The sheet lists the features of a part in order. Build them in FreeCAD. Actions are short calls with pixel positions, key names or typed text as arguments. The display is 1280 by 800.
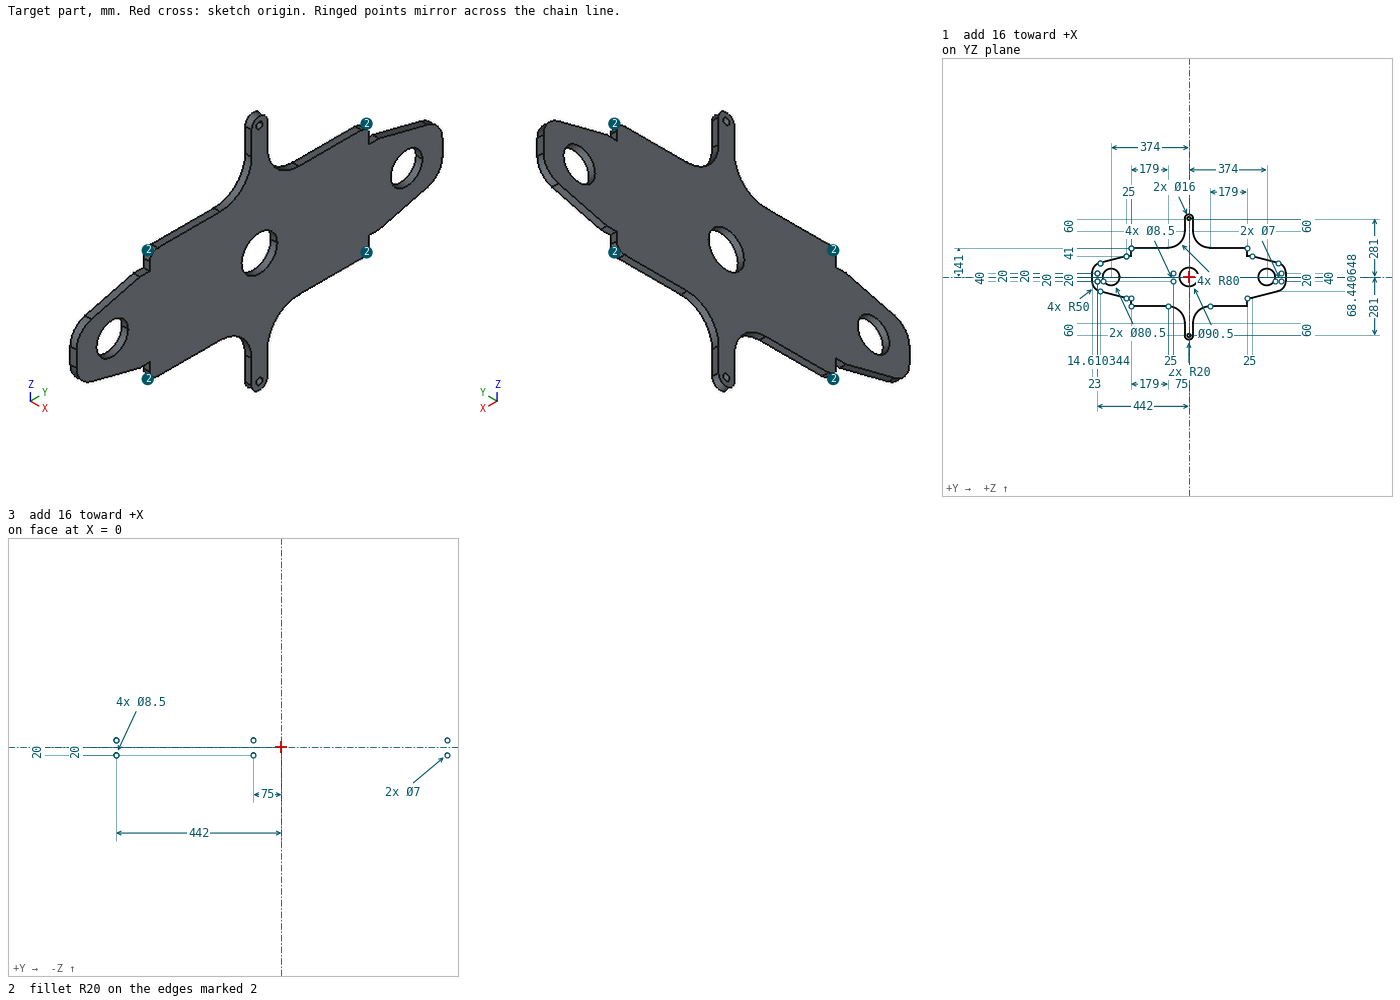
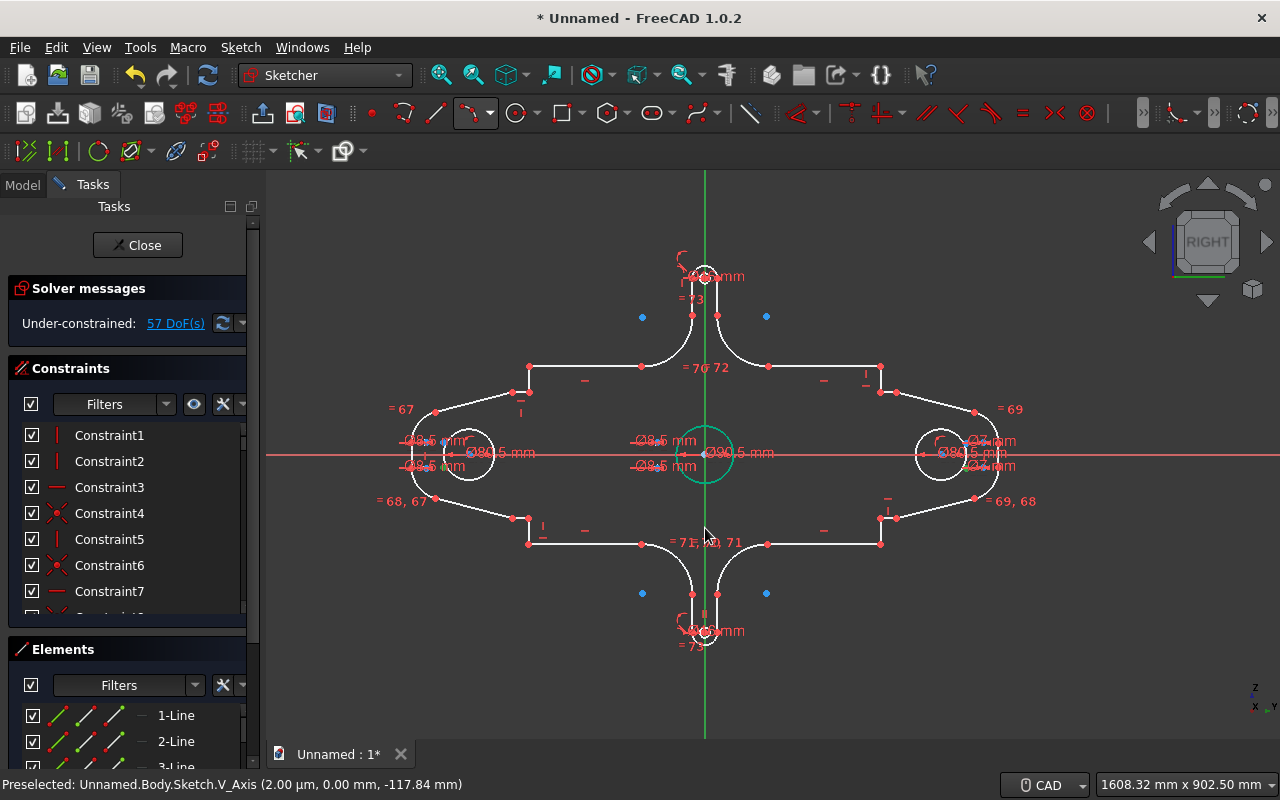
click(1056, 114)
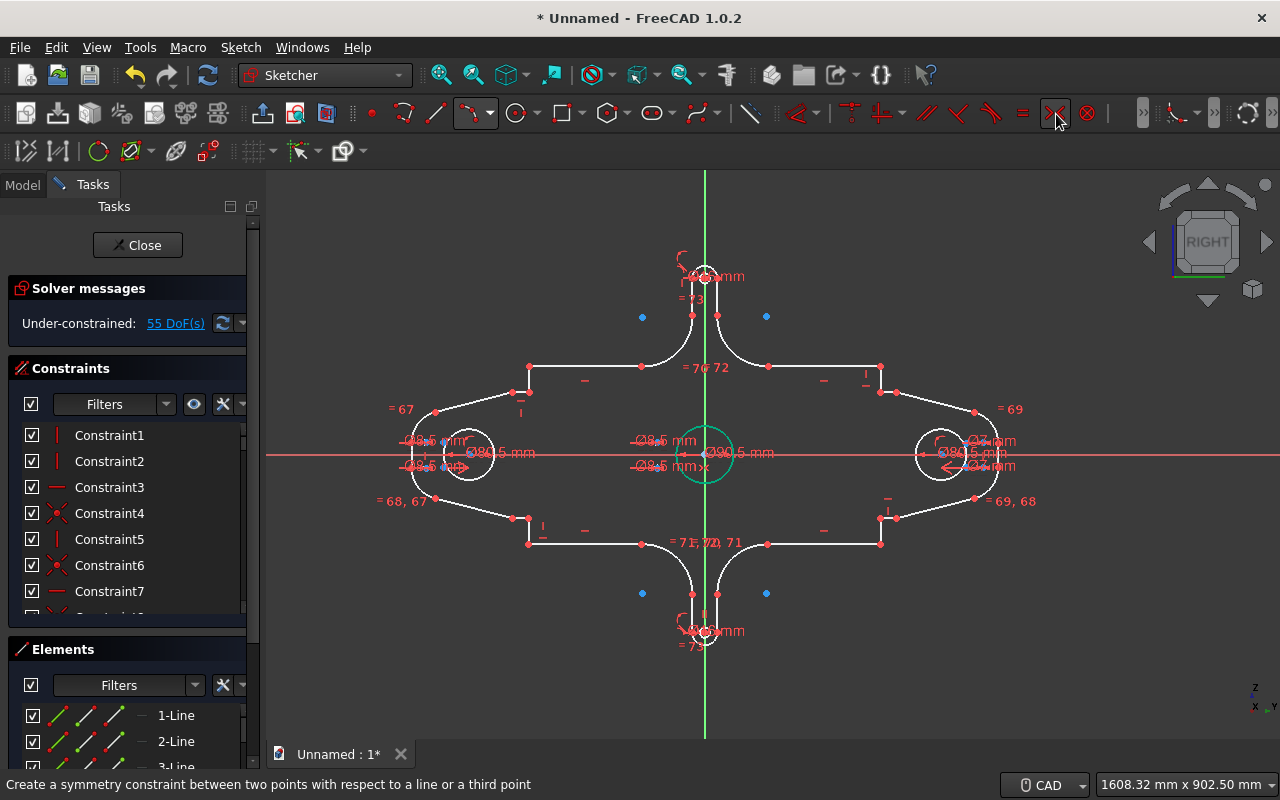
click(426, 468)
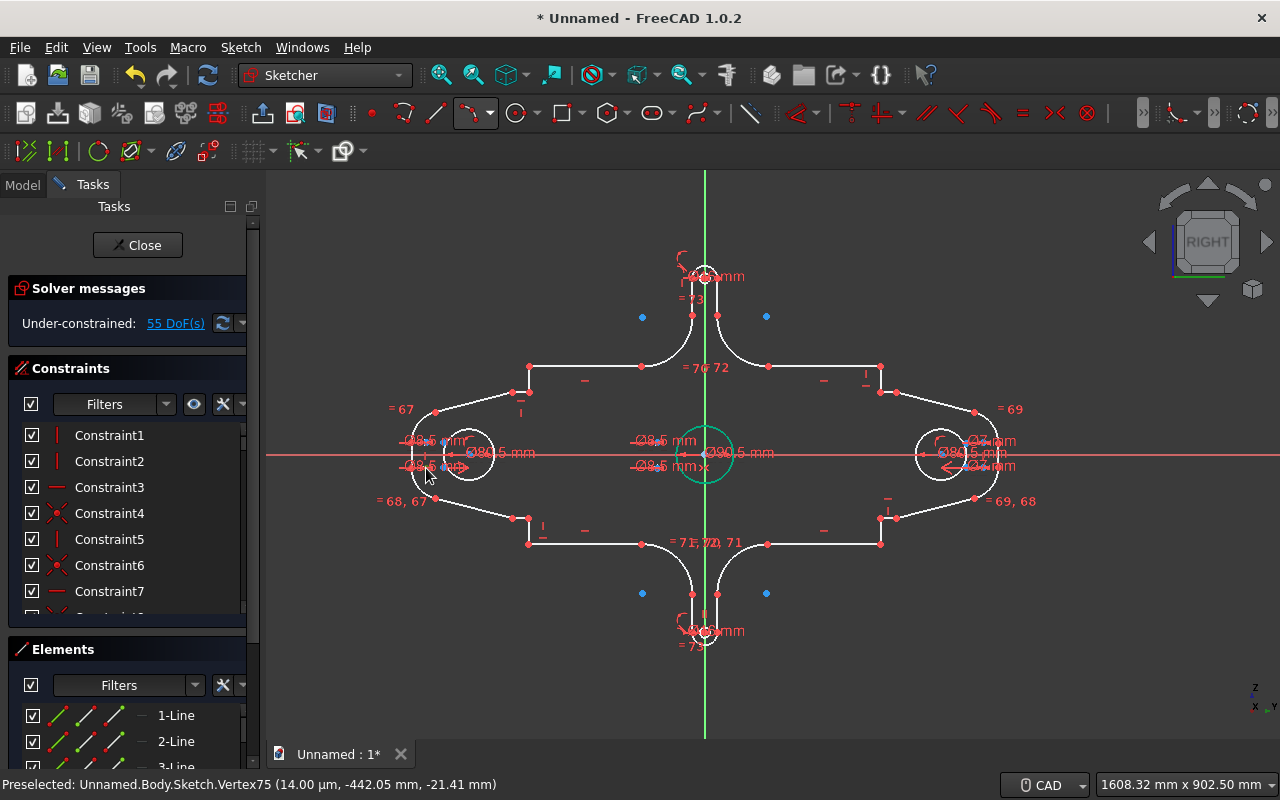
click(426, 443)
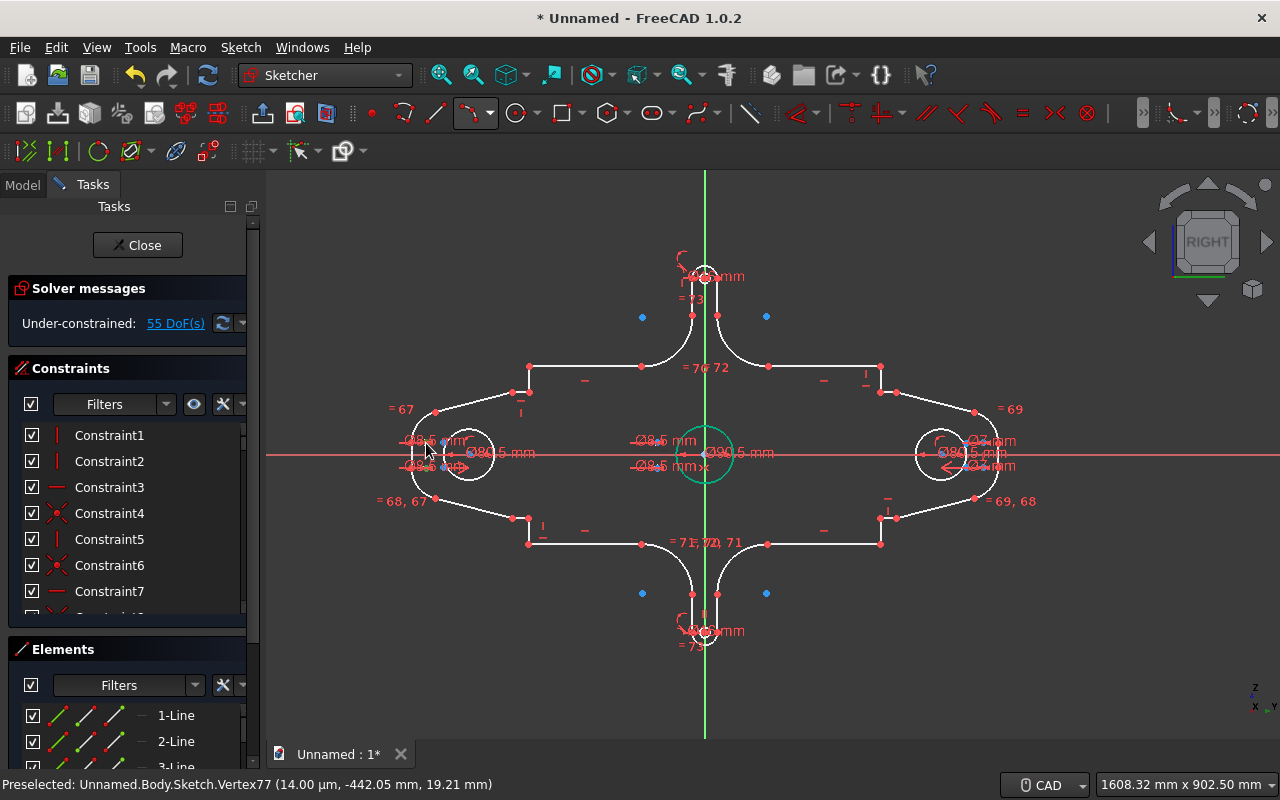
click(353, 455)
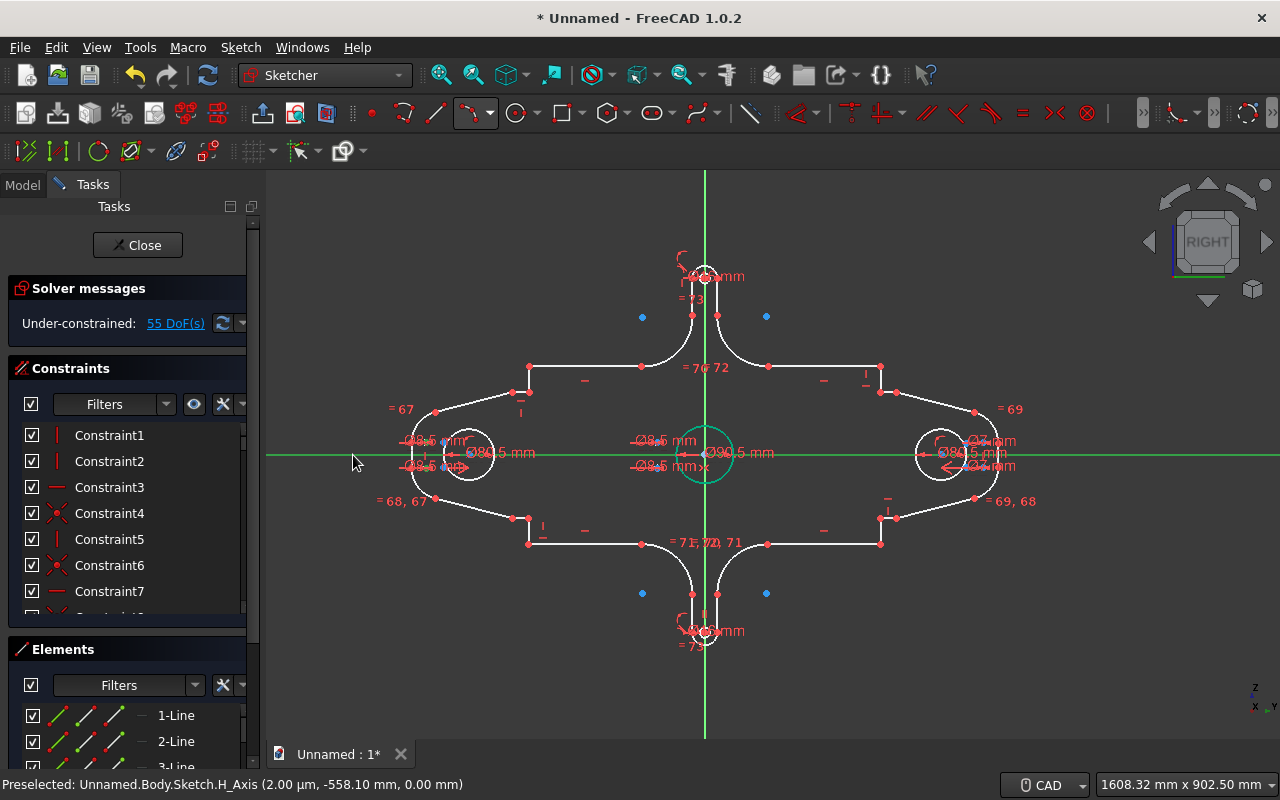
click(1056, 114)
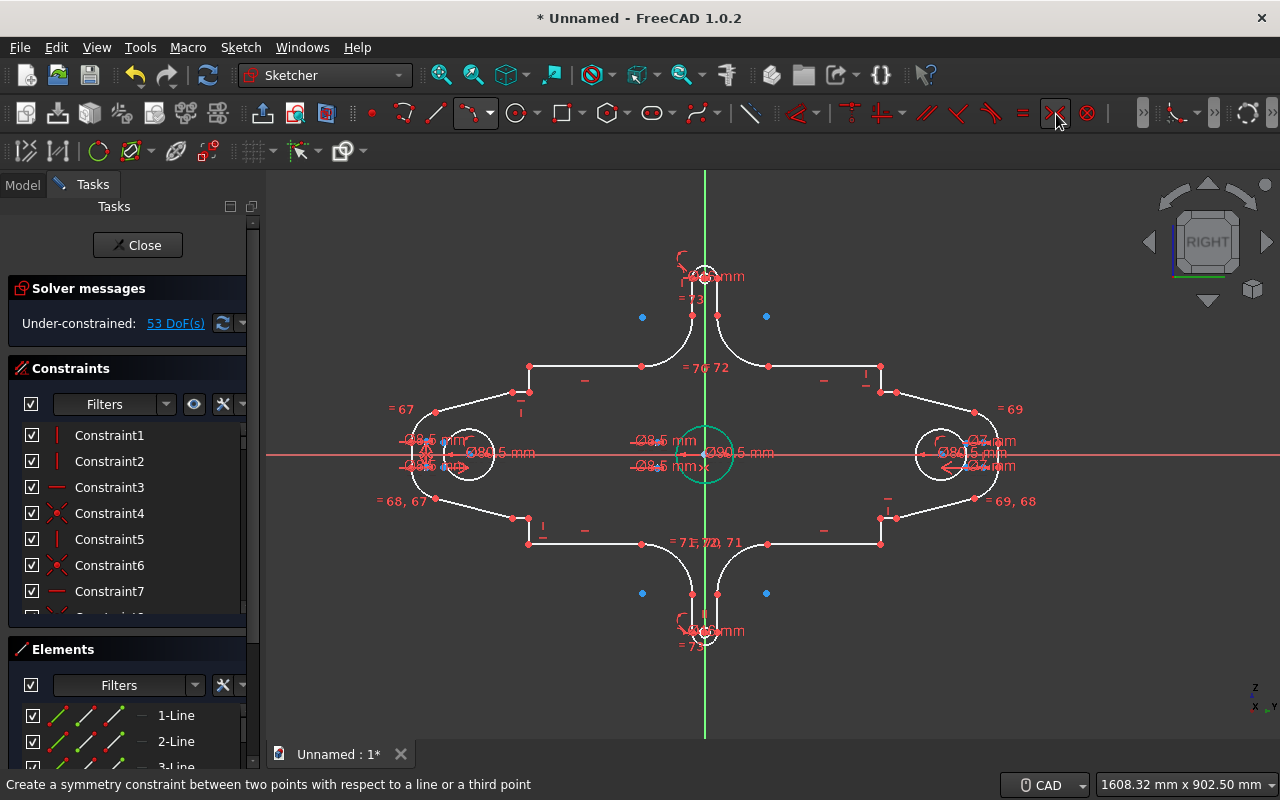
click(657, 468)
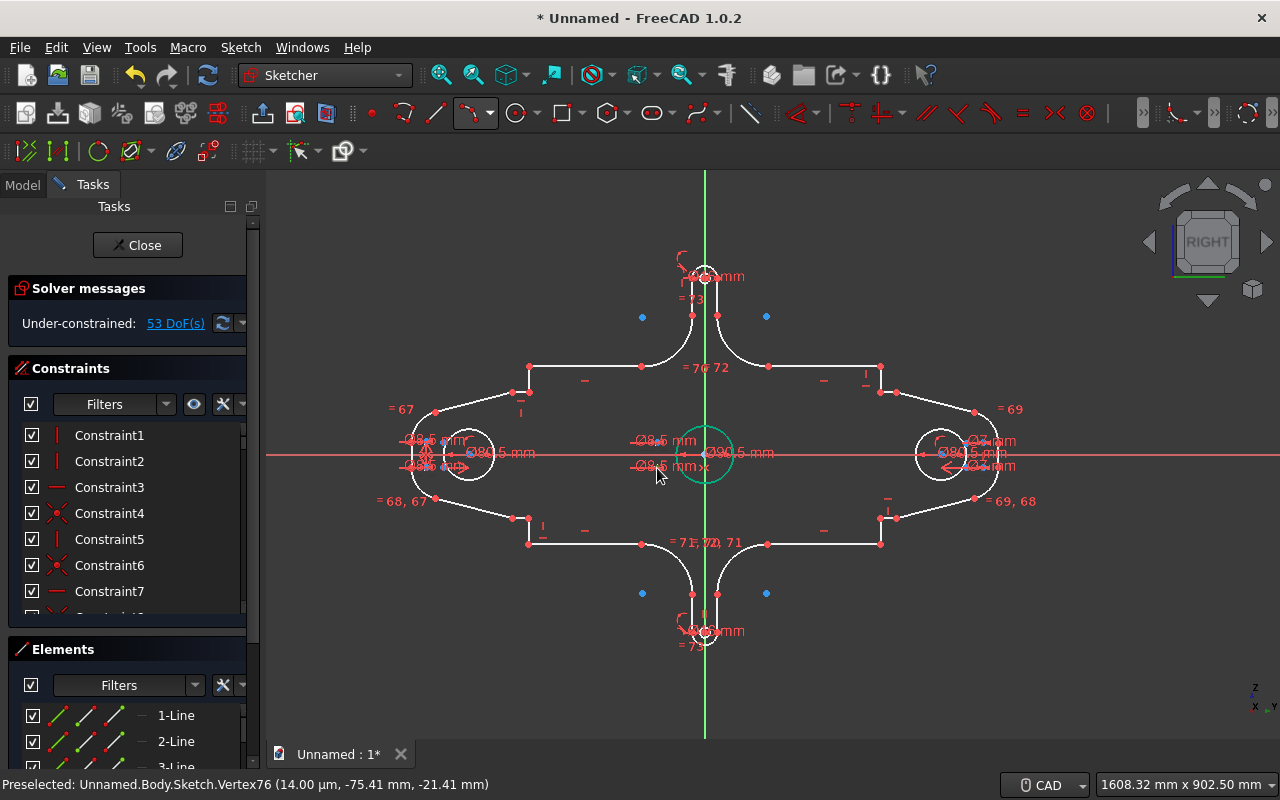
click(657, 443)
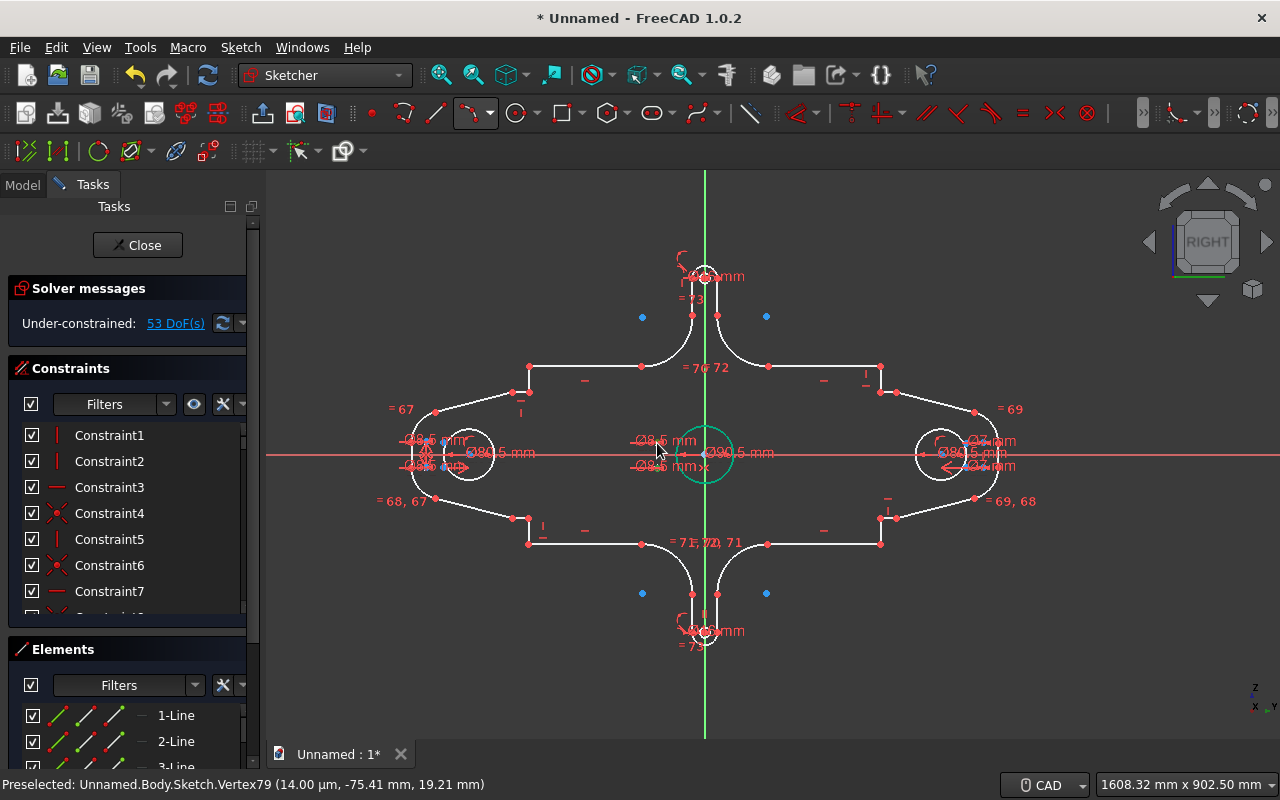
click(353, 455)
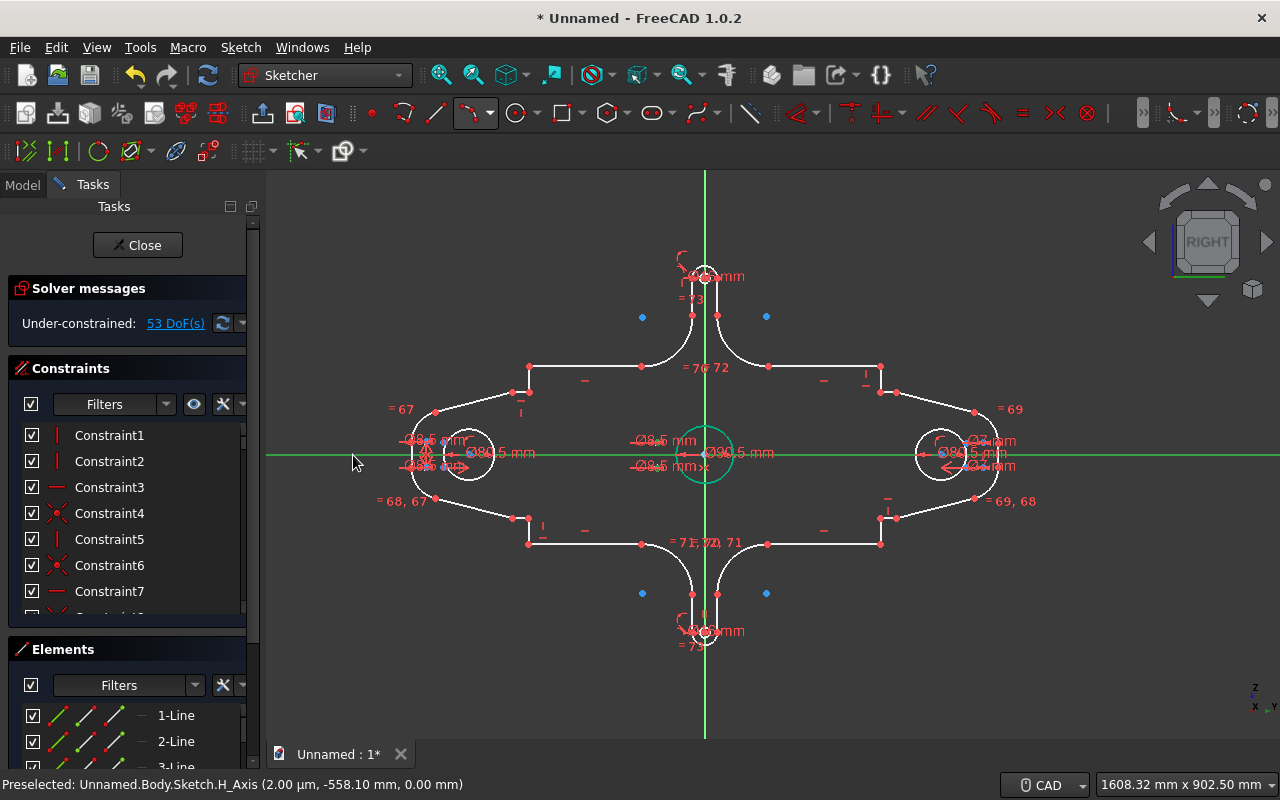
click(1056, 114)